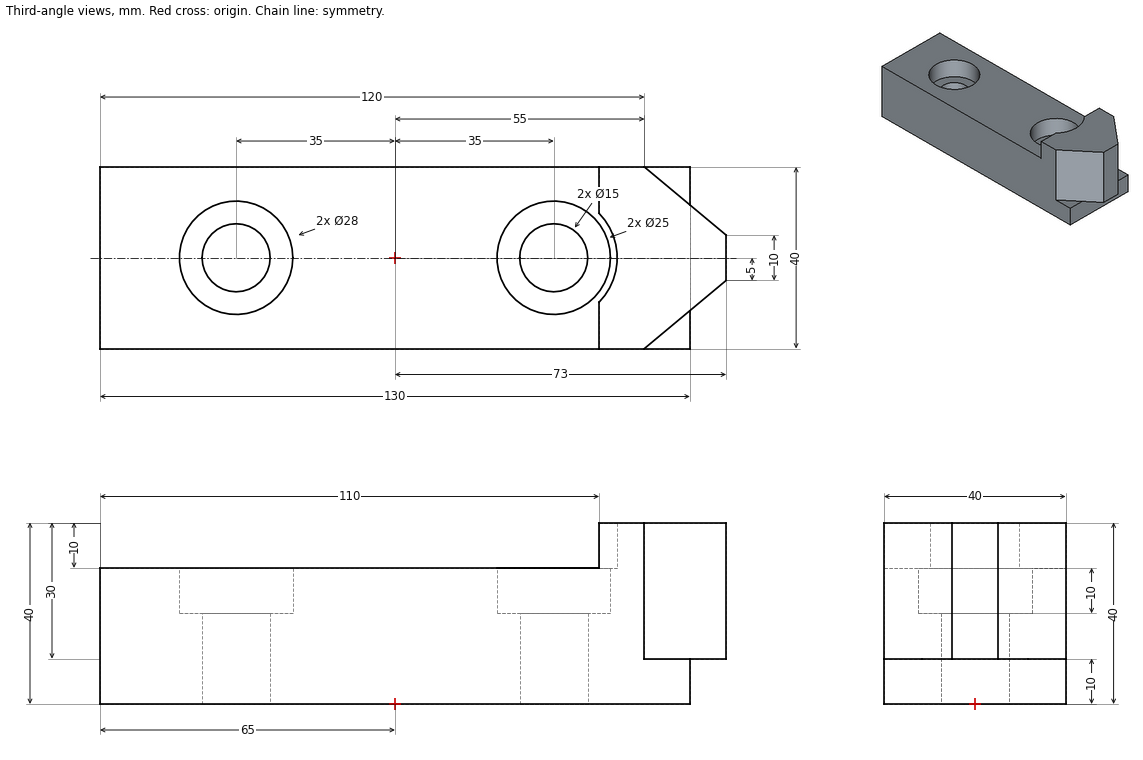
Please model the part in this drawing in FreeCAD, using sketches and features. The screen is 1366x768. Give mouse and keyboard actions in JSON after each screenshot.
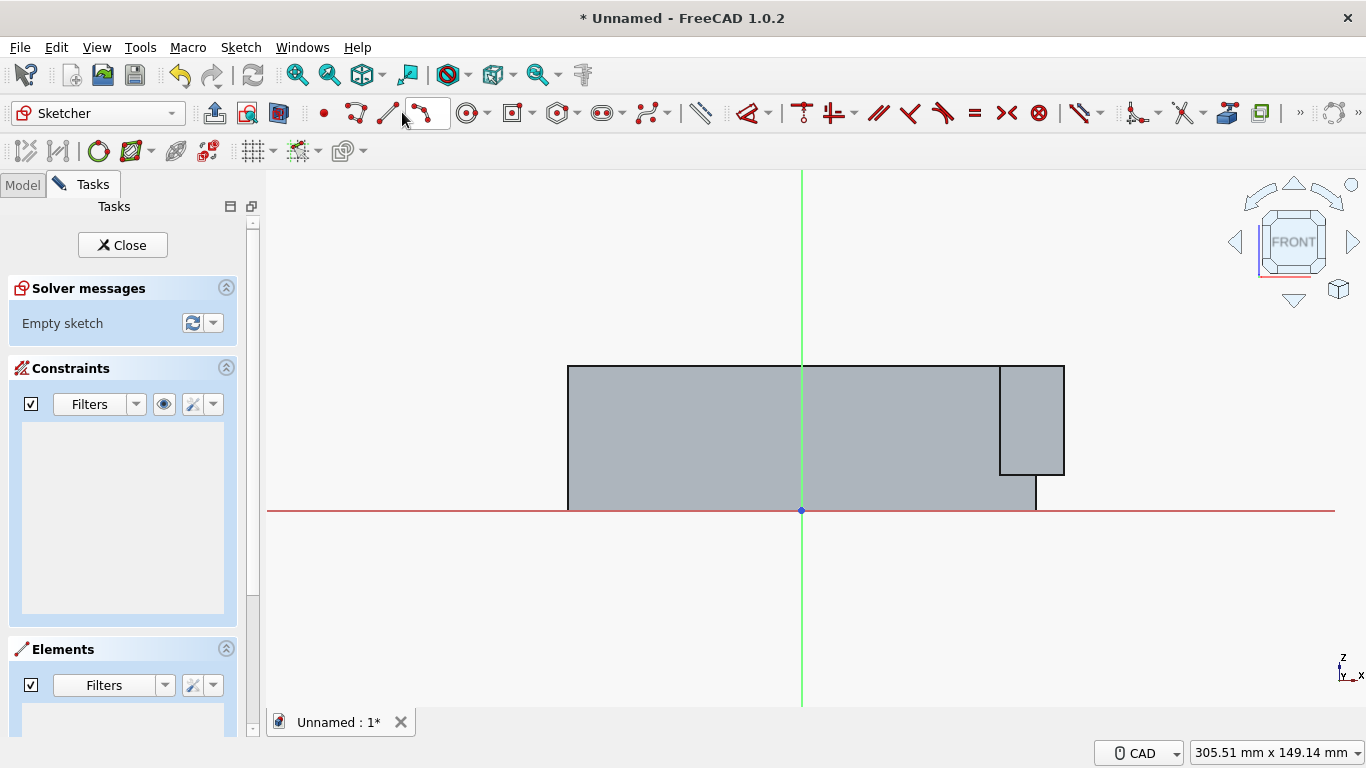
{"action": "scroll", "coordinate": [802, 439], "scroll_direction": "up", "scroll_amount": 2}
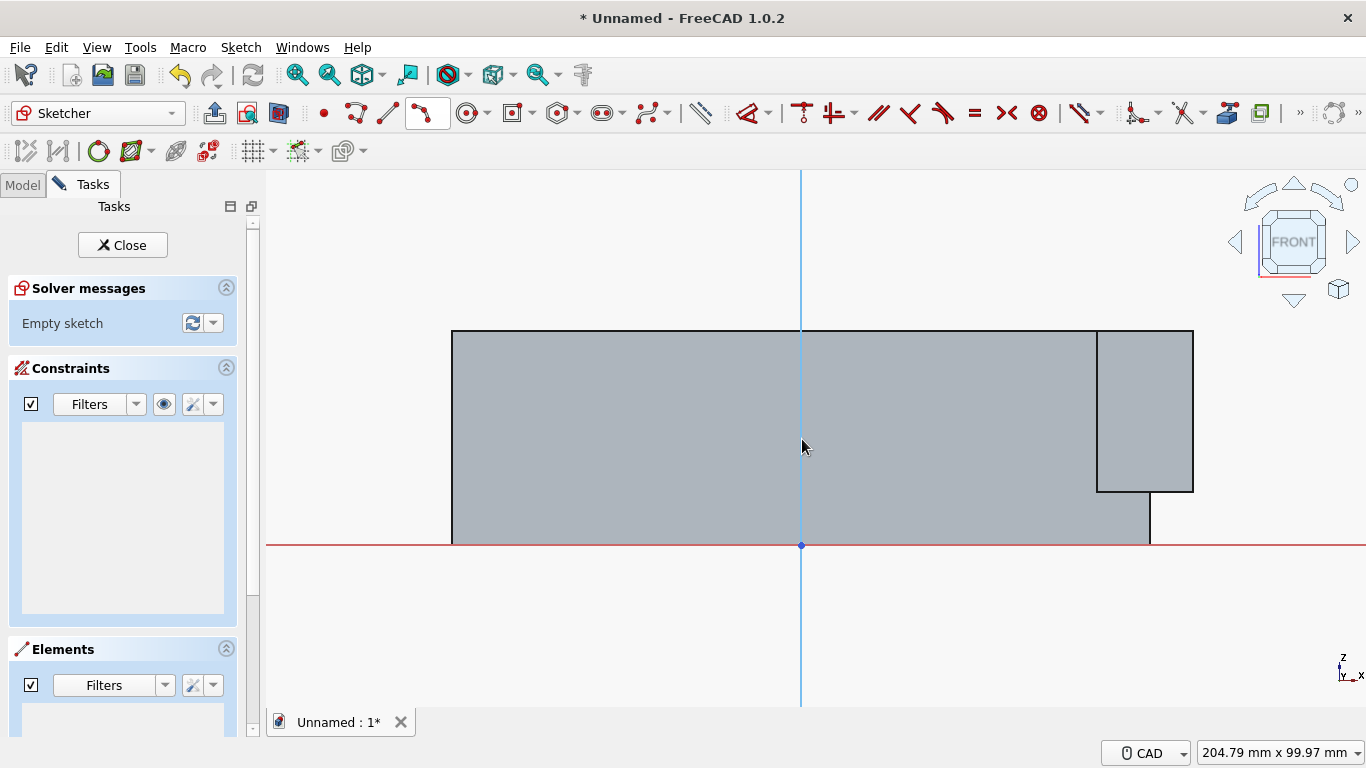
{"action": "left_click", "coordinate": [534, 114]}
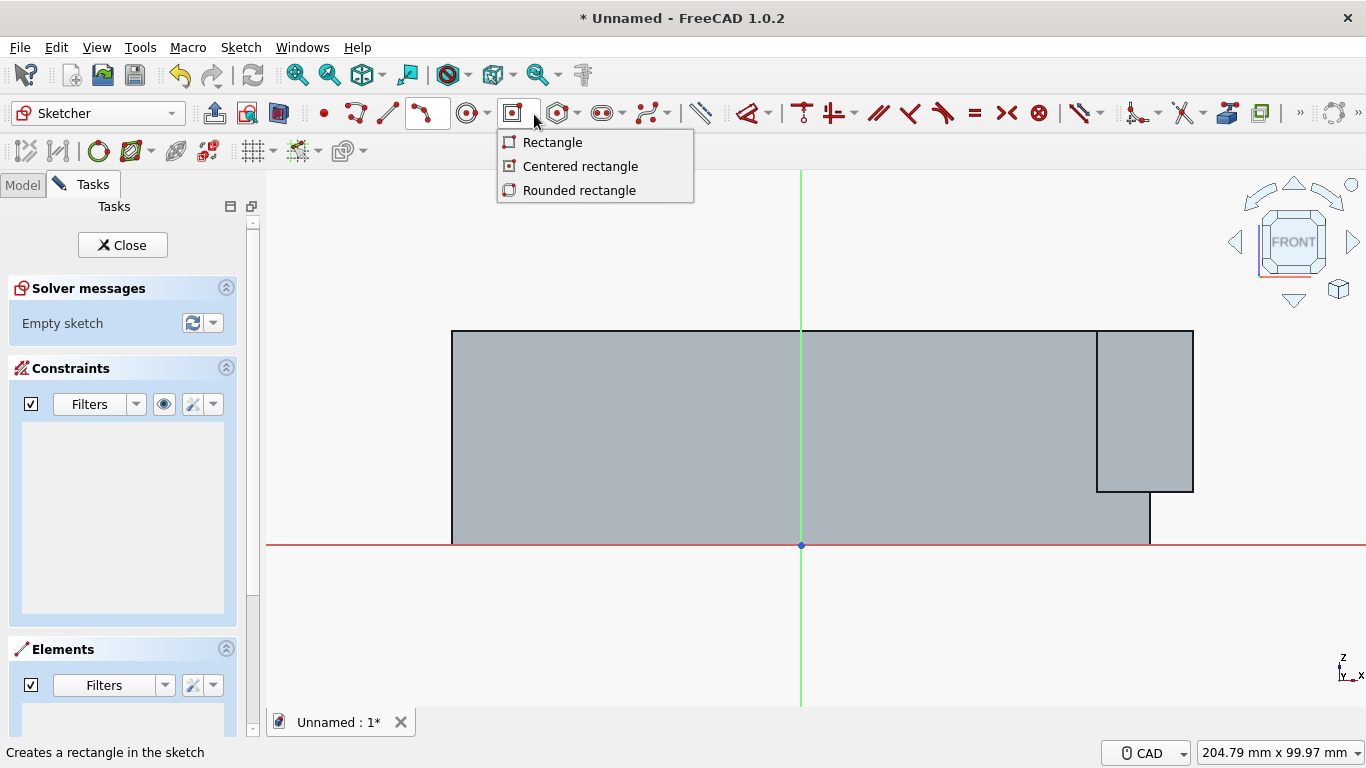
{"action": "left_click", "coordinate": [596, 142]}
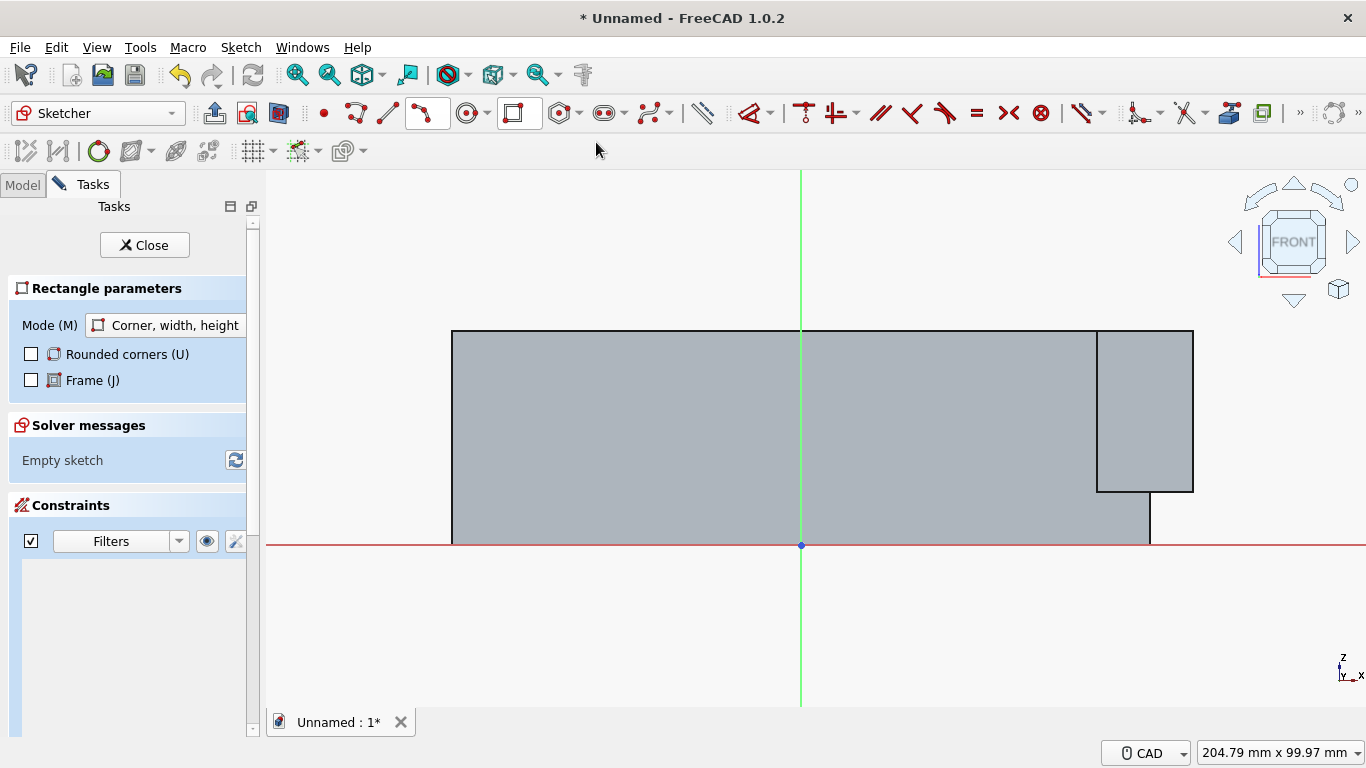
{"action": "left_click", "coordinate": [452, 331]}
{"action": "left_click", "coordinate": [1043, 384]}
{"action": "key", "text": "Escape"}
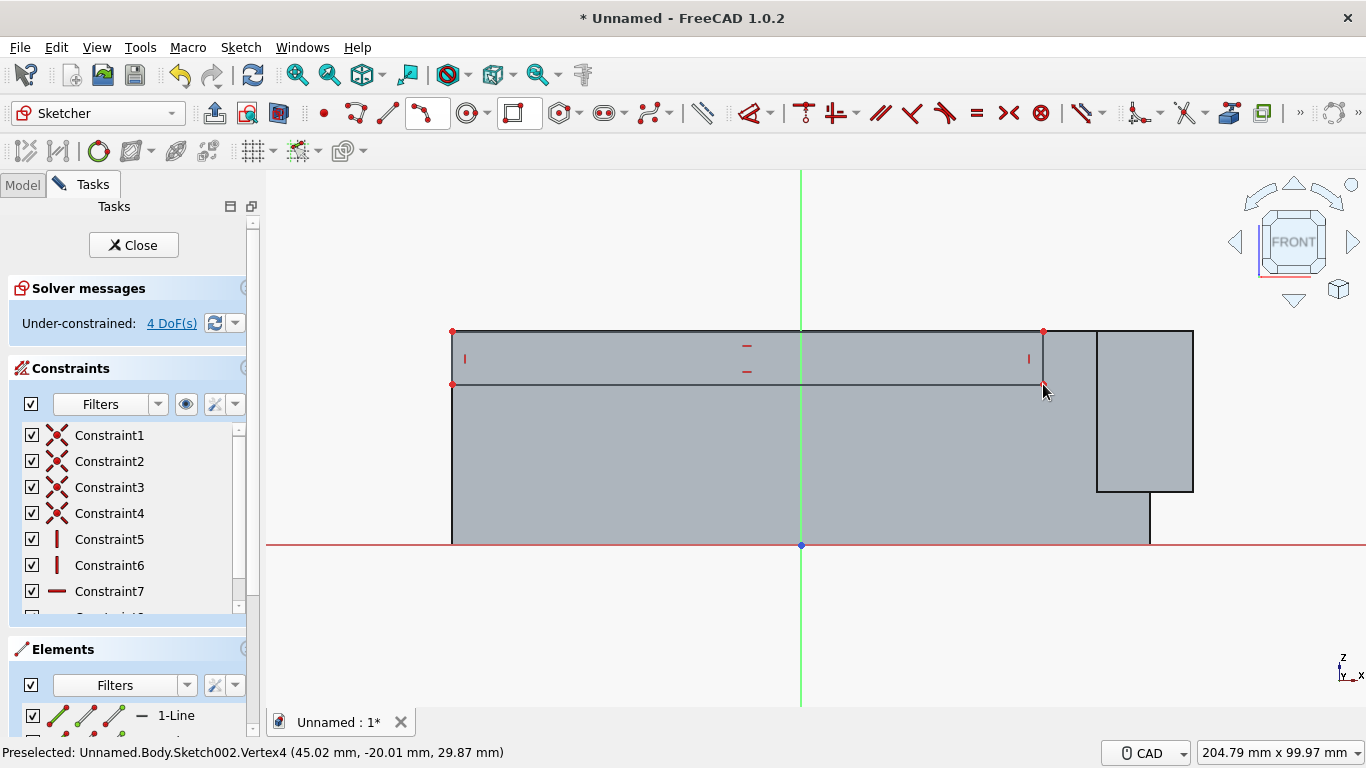
{"action": "left_click", "coordinate": [750, 114]}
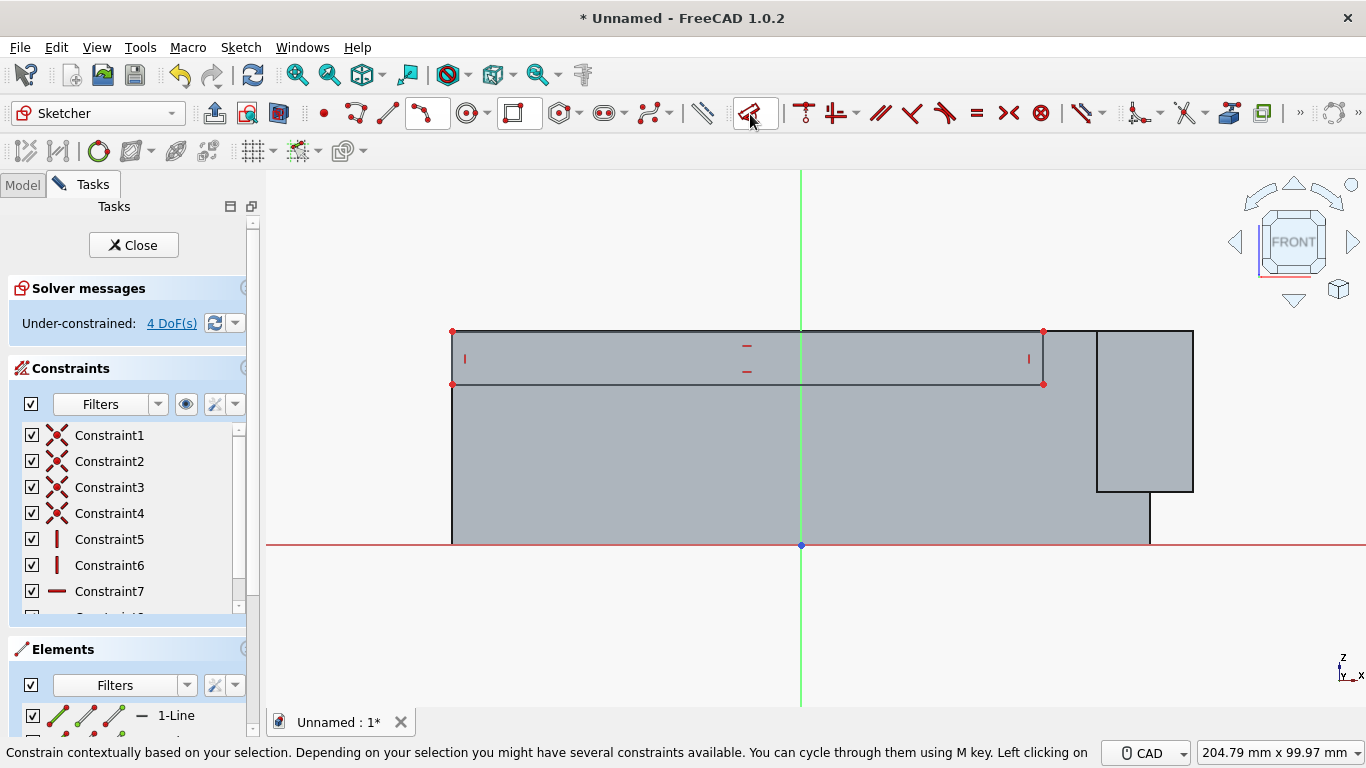
{"action": "left_click", "coordinate": [452, 348]}
{"action": "left_click", "coordinate": [418, 359]}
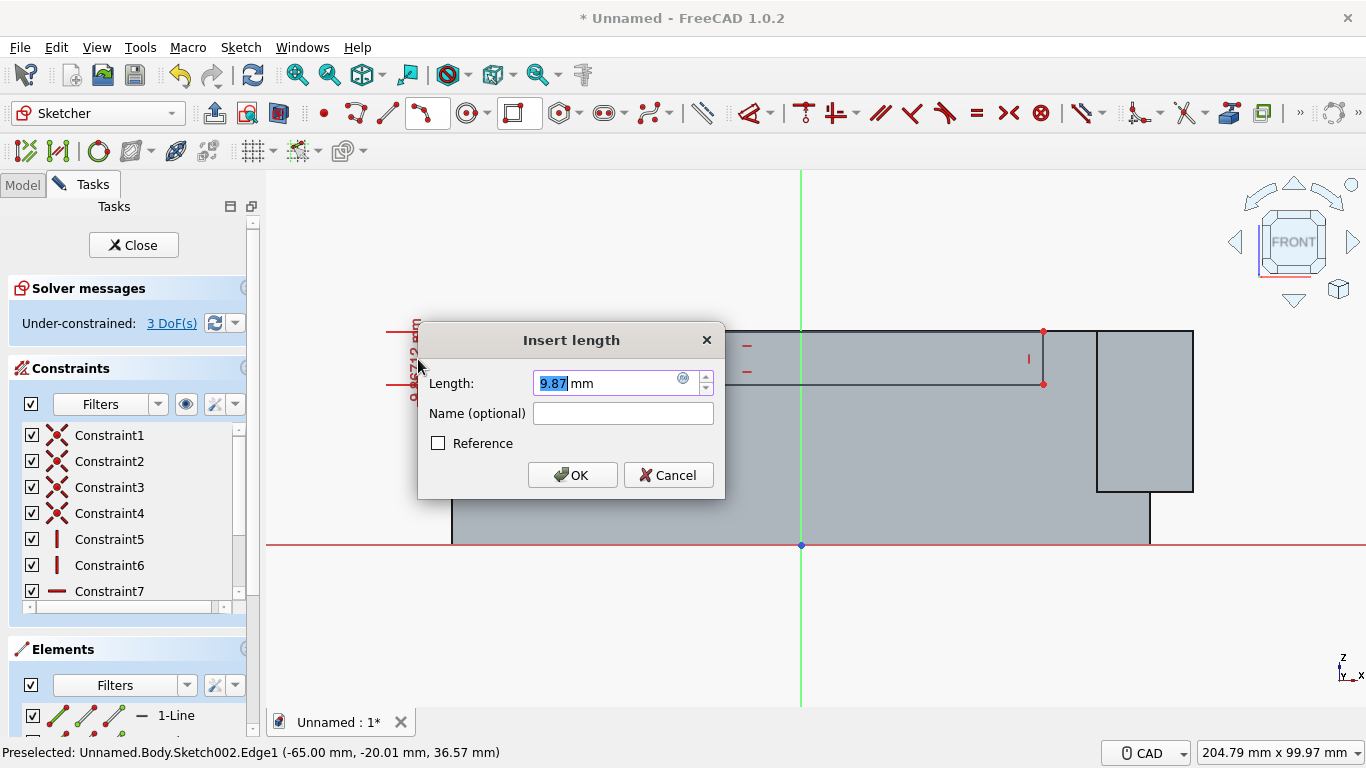
{"action": "type", "text": "10"}
{"action": "key", "text": "Return"}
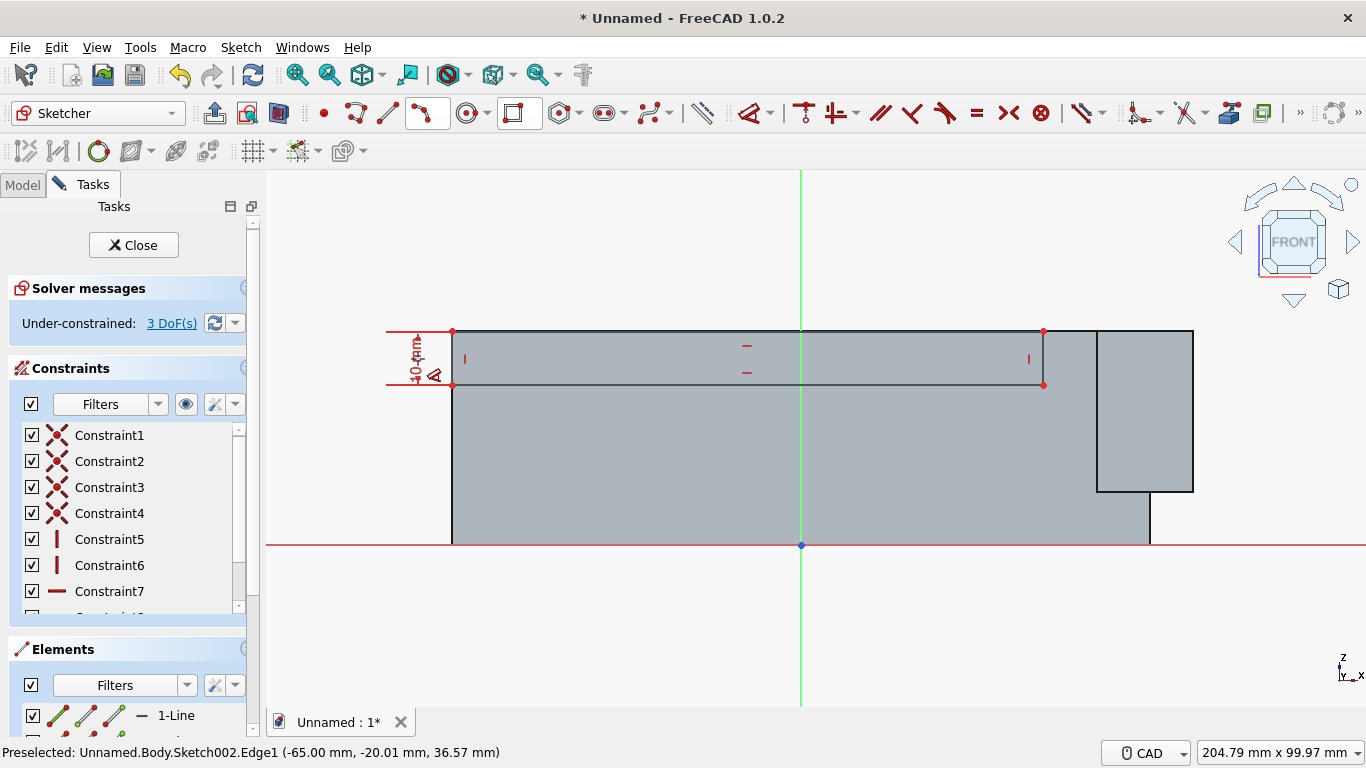
{"action": "left_click", "coordinate": [629, 385]}
{"action": "left_click", "coordinate": [747, 351]}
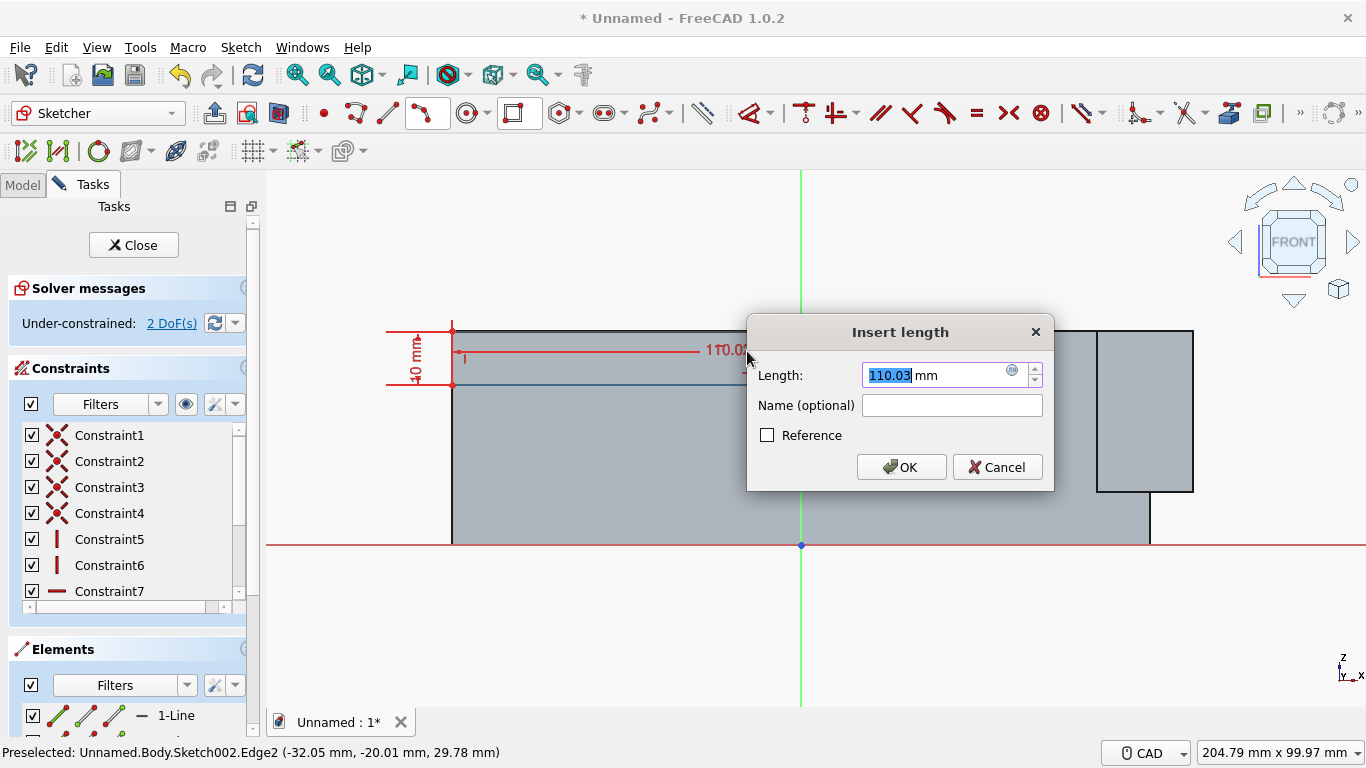
{"action": "type", "text": "110"}
{"action": "key", "text": "Return"}